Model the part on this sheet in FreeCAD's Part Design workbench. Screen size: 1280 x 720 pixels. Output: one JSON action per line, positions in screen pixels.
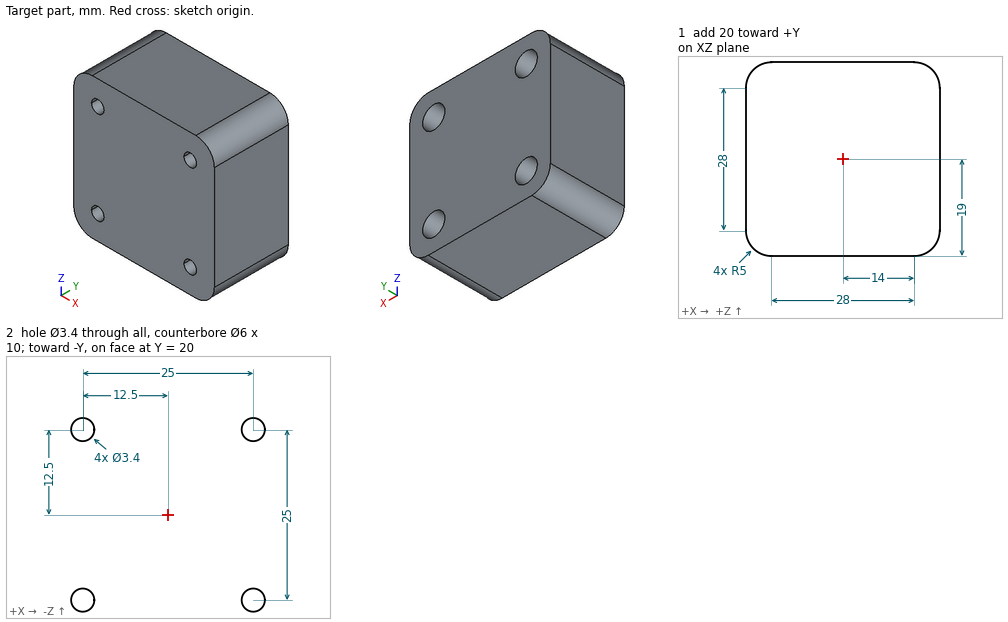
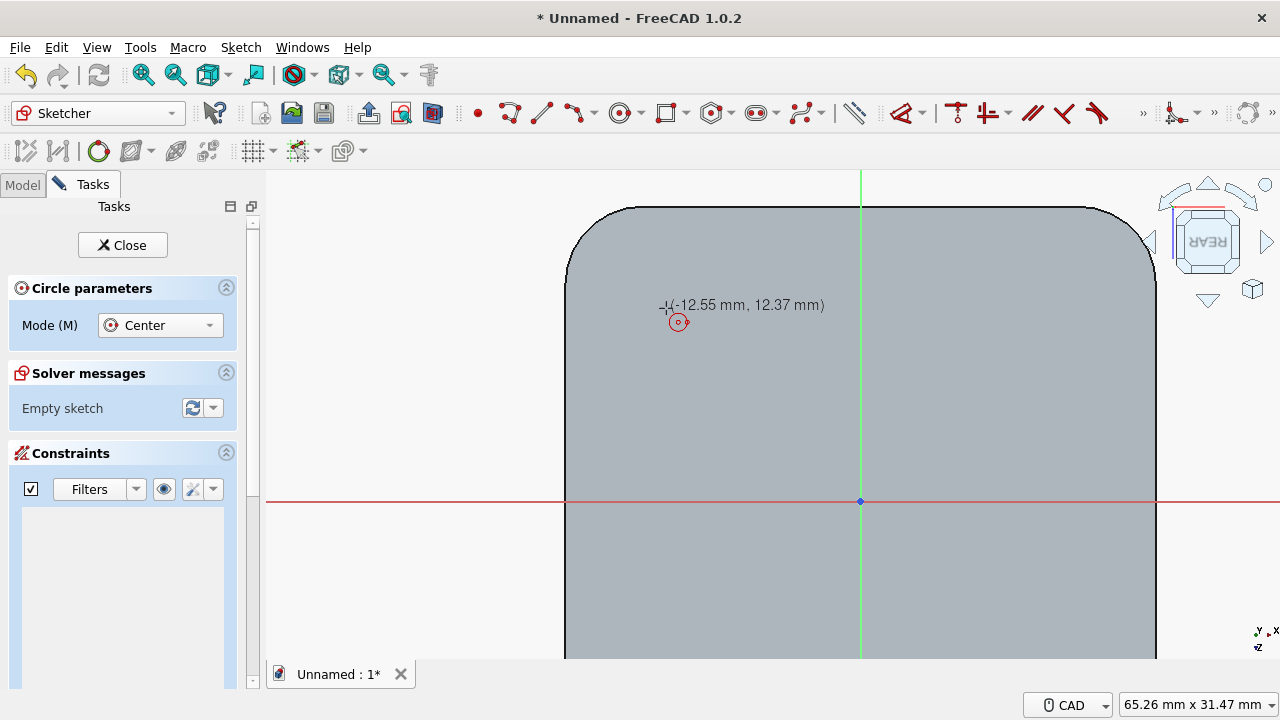
{"action": "left_click", "coordinate": [666, 308]}
{"action": "left_click", "coordinate": [685, 289]}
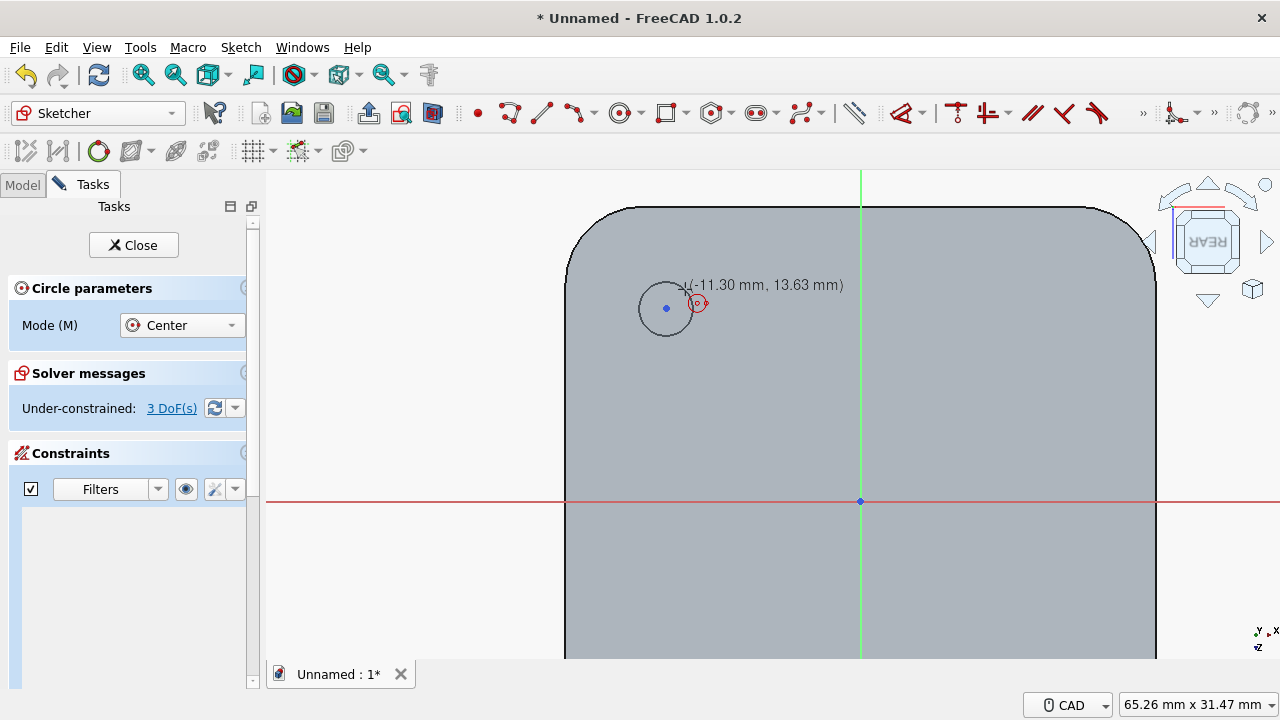
{"action": "left_click", "coordinate": [1055, 308]}
{"action": "left_click", "coordinate": [1074, 289]}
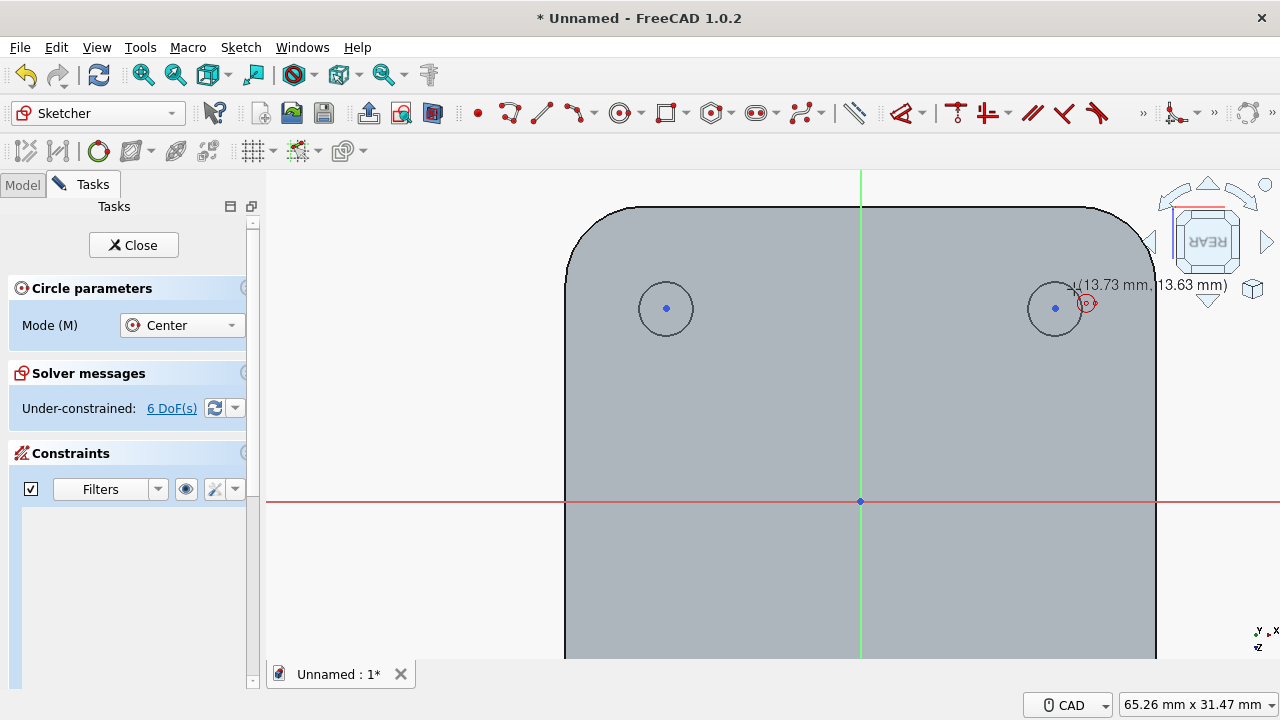
{"action": "scroll", "coordinate": [387, 237], "scroll_direction": "down", "scroll_amount": 2}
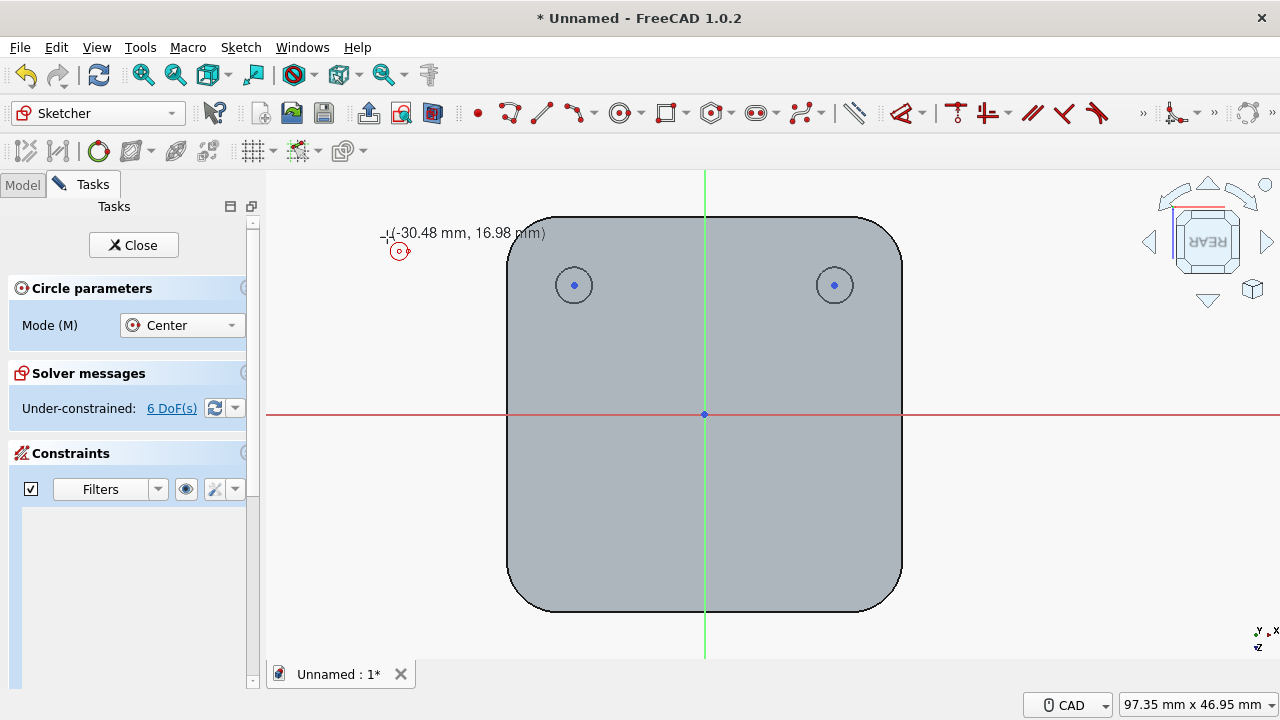
{"action": "scroll", "coordinate": [835, 545], "scroll_direction": "up", "scroll_amount": 2}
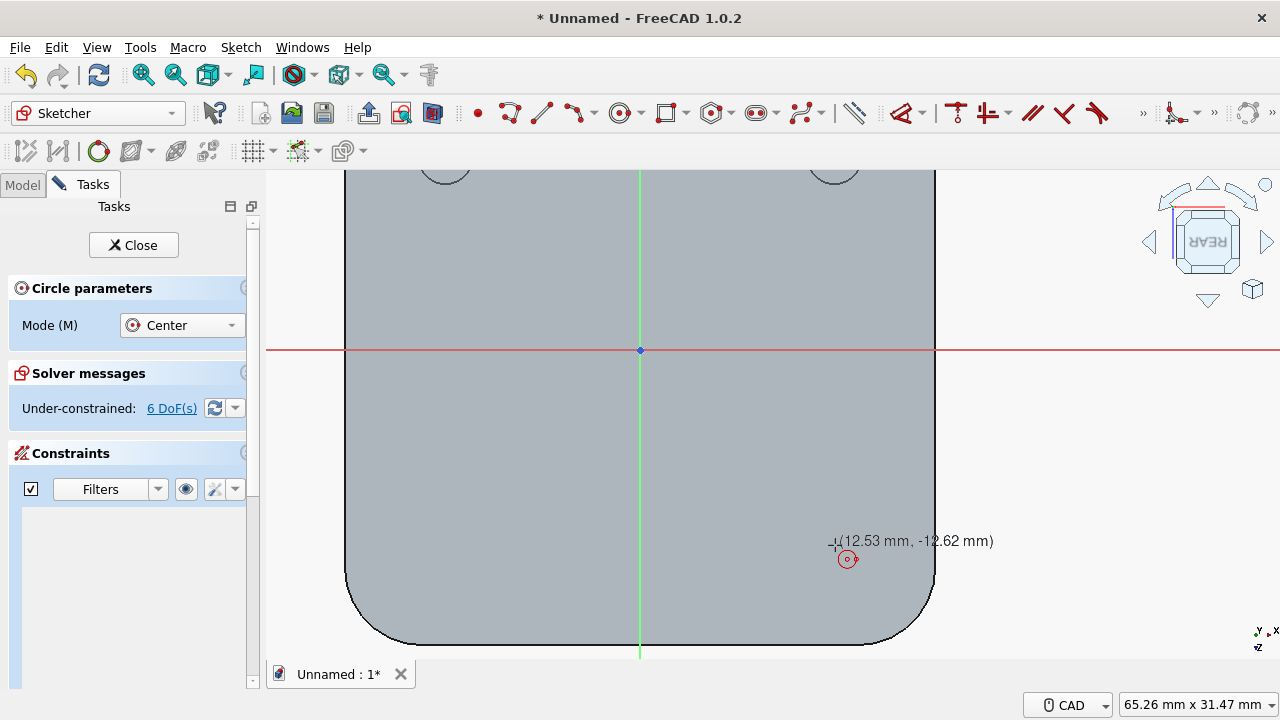
{"action": "left_click", "coordinate": [834, 544]}
{"action": "left_click", "coordinate": [853, 526]}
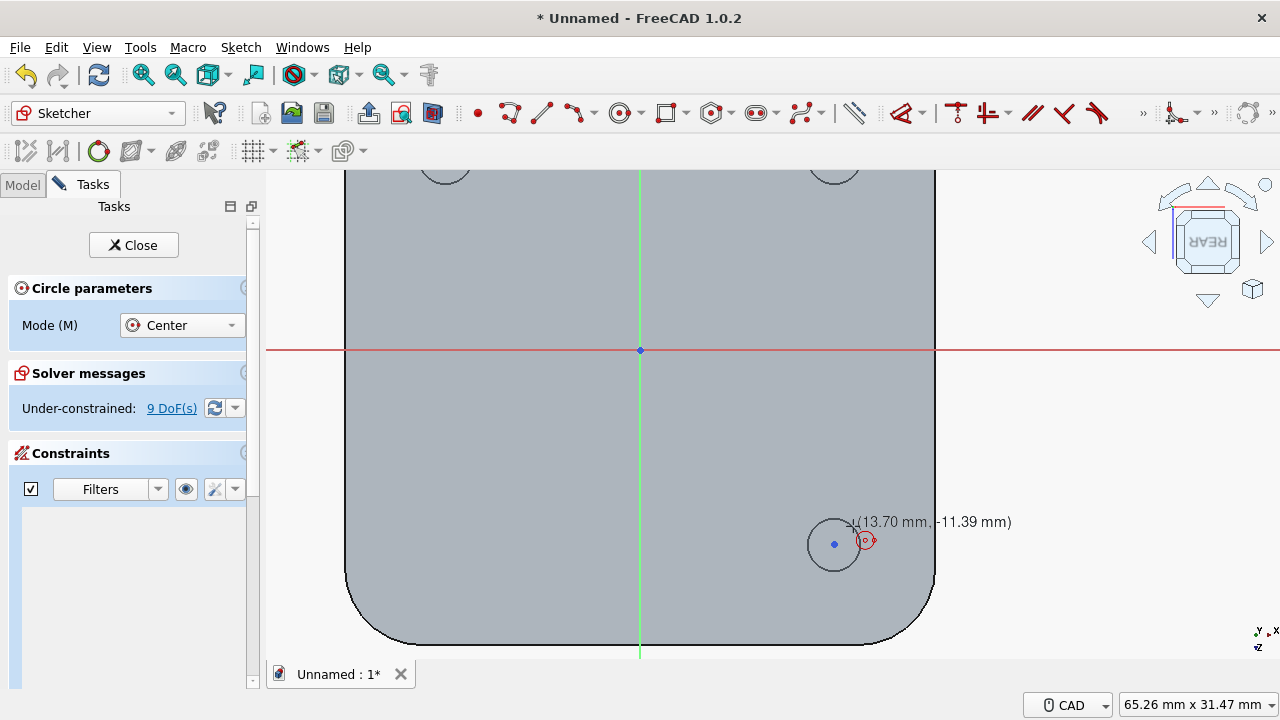
{"action": "left_click", "coordinate": [446, 544]}
{"action": "left_click", "coordinate": [465, 526]}
{"action": "key", "text": "Escape"}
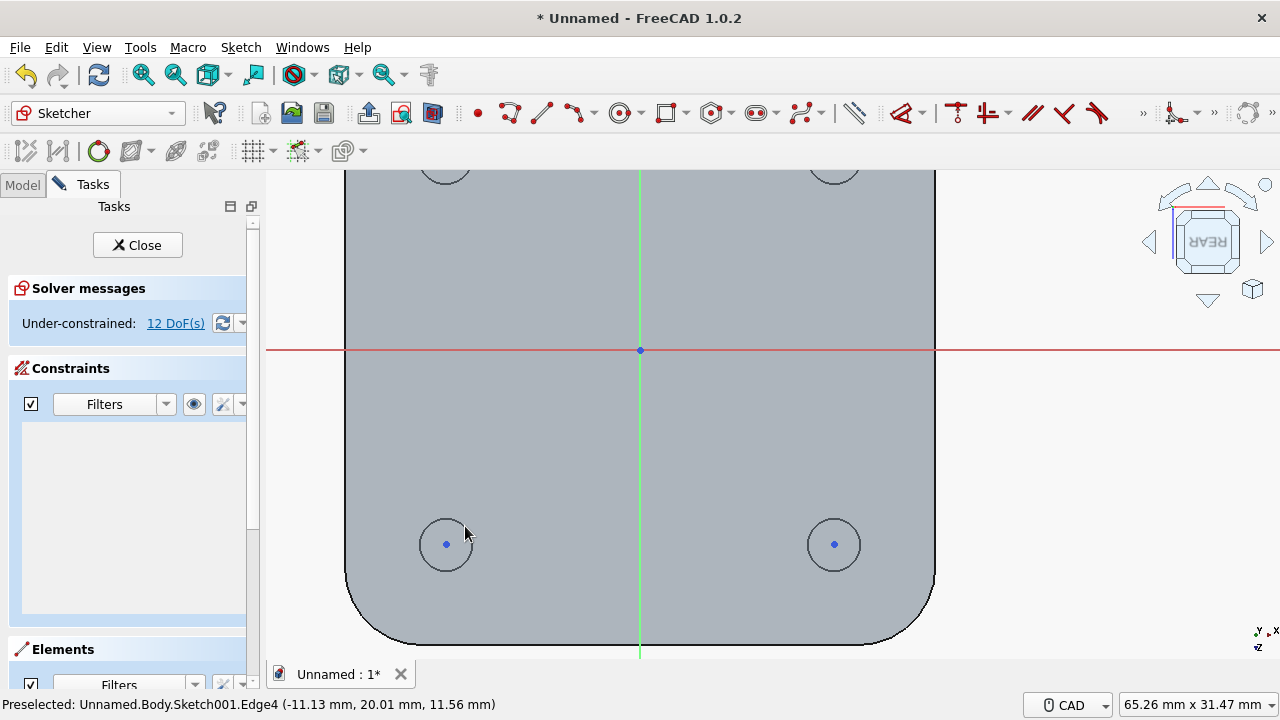
{"action": "scroll", "coordinate": [835, 546], "scroll_direction": "down", "scroll_amount": 2}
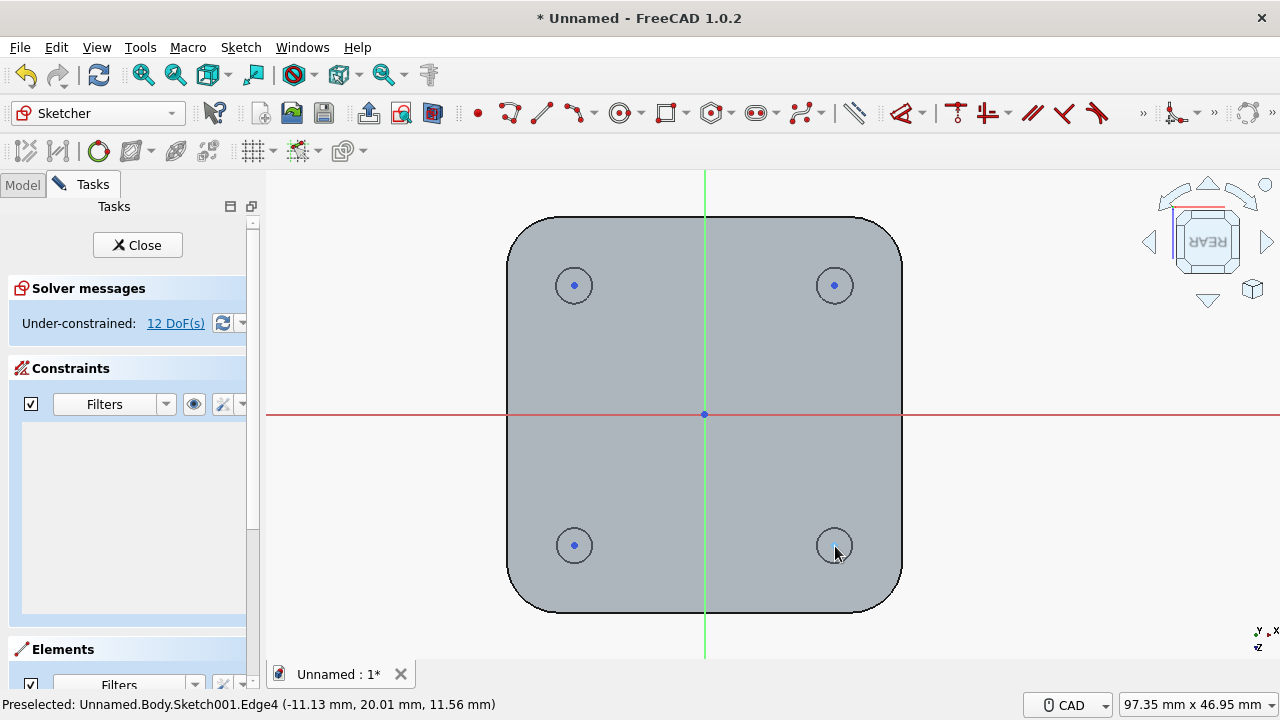
{"action": "left_click", "coordinate": [587, 273]}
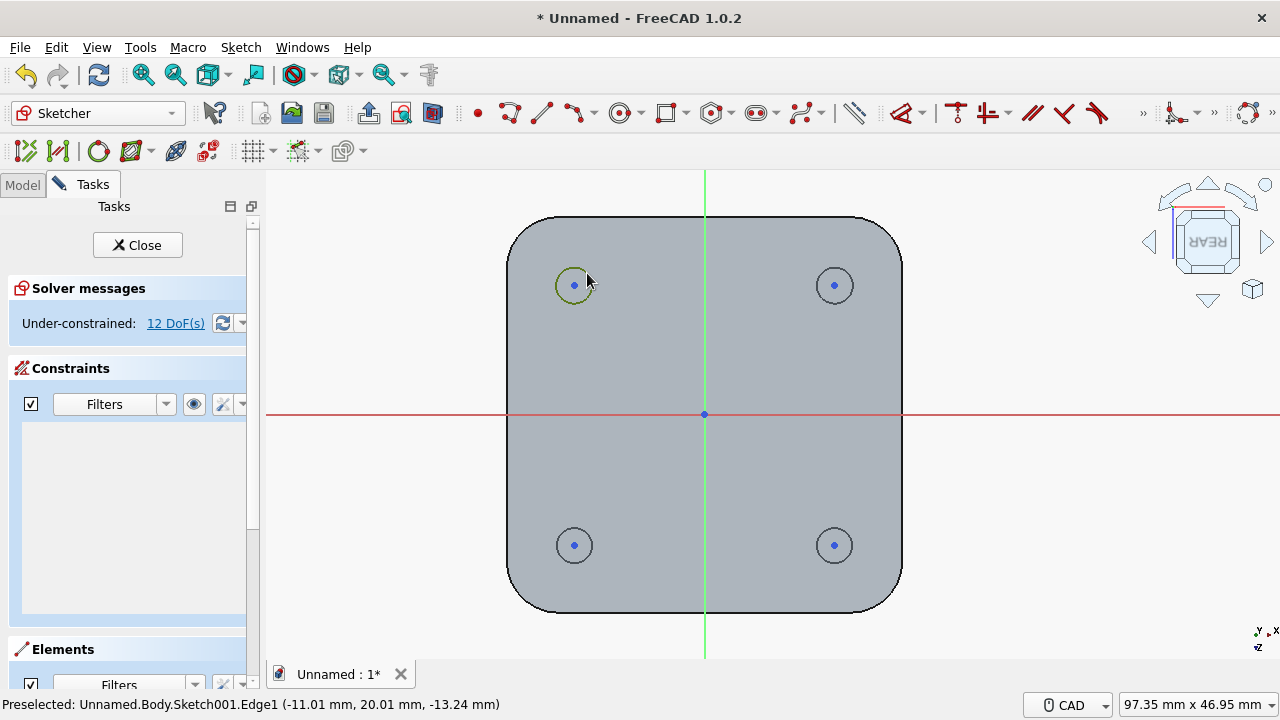
{"action": "left_click", "coordinate": [848, 273]}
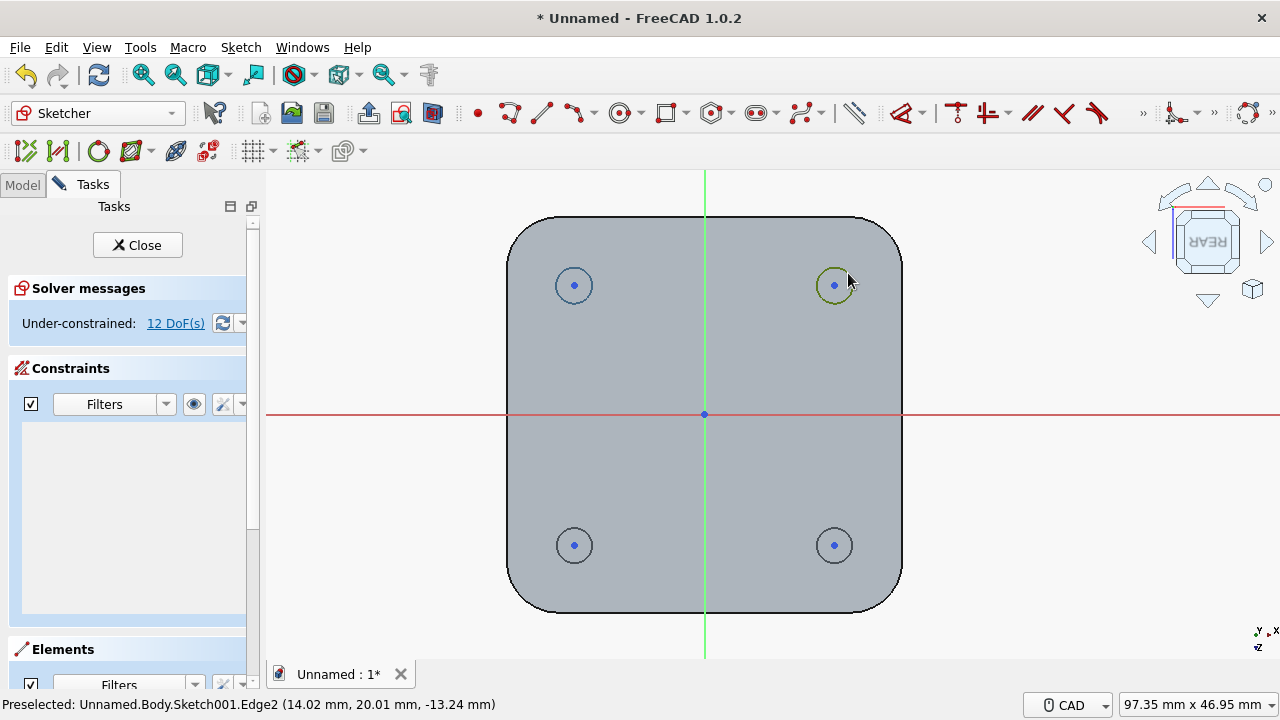
{"action": "left_click", "coordinate": [847, 533]}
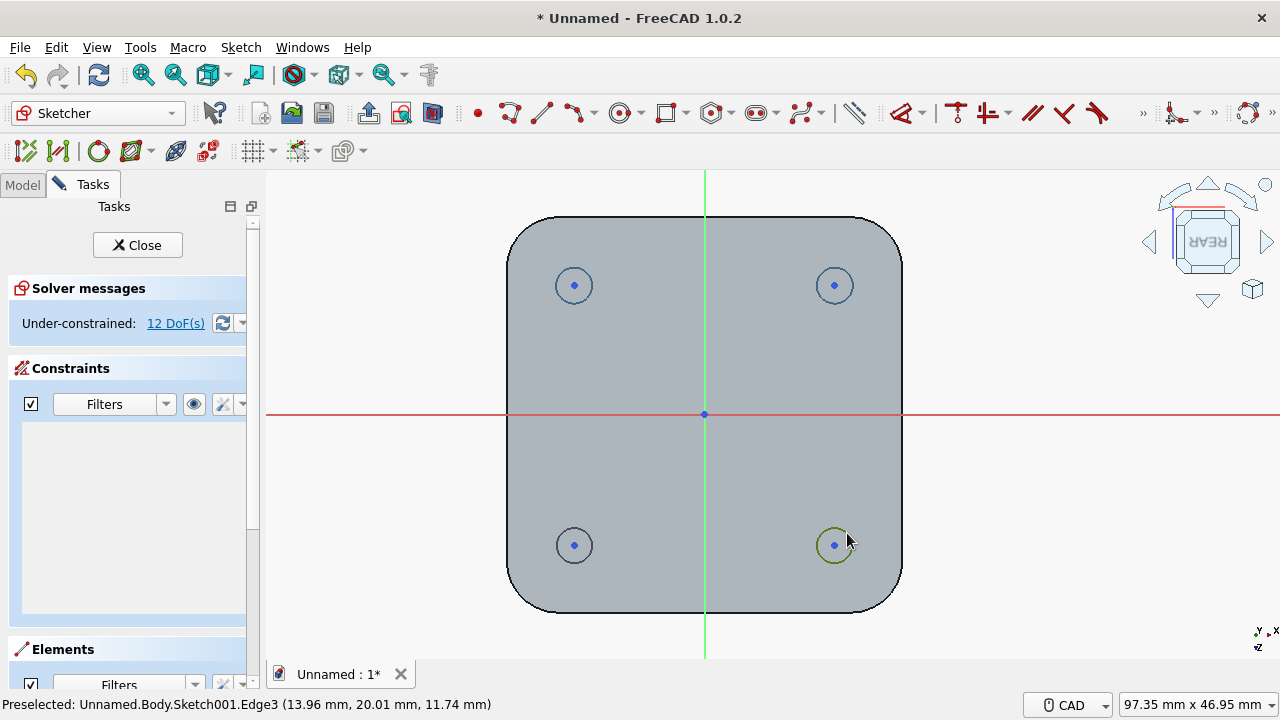
{"action": "left_click", "coordinate": [587, 533]}